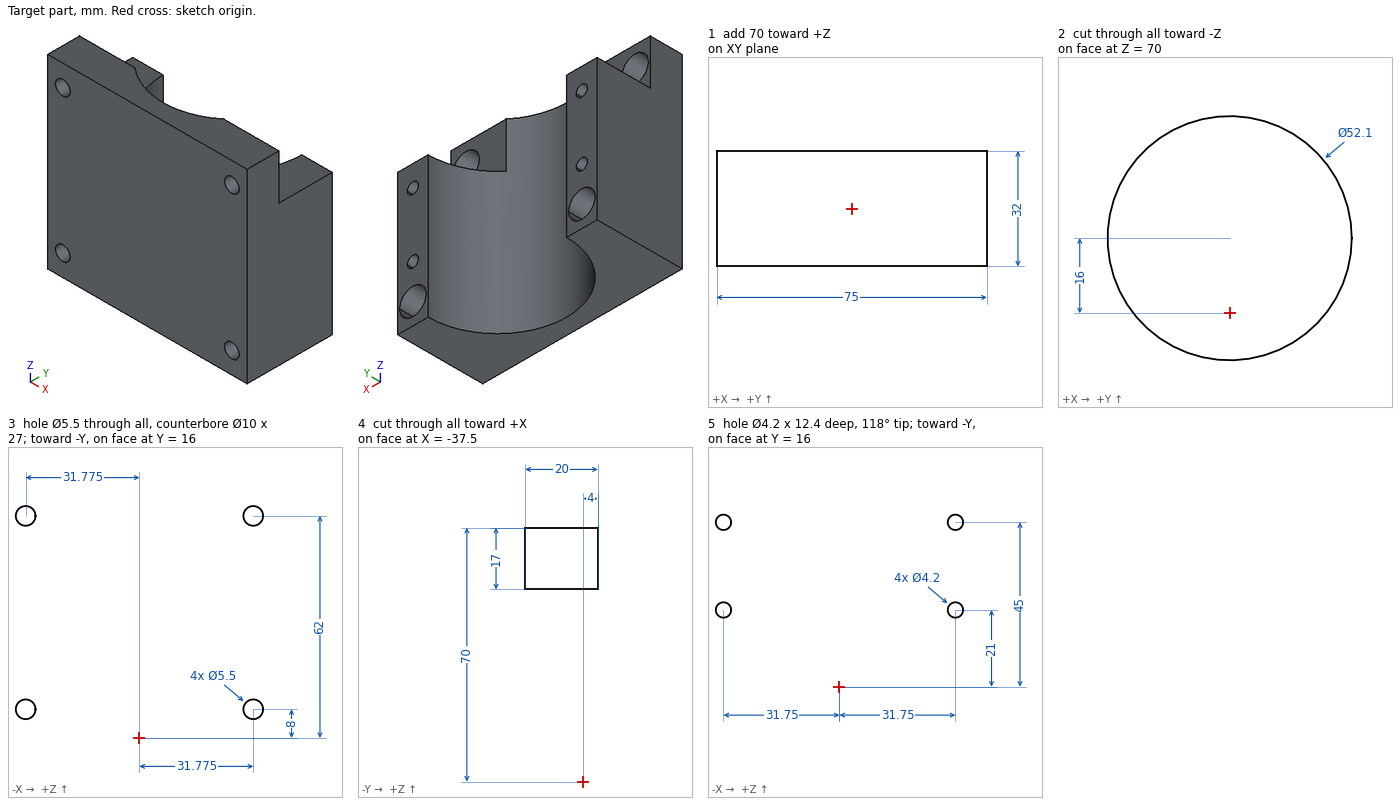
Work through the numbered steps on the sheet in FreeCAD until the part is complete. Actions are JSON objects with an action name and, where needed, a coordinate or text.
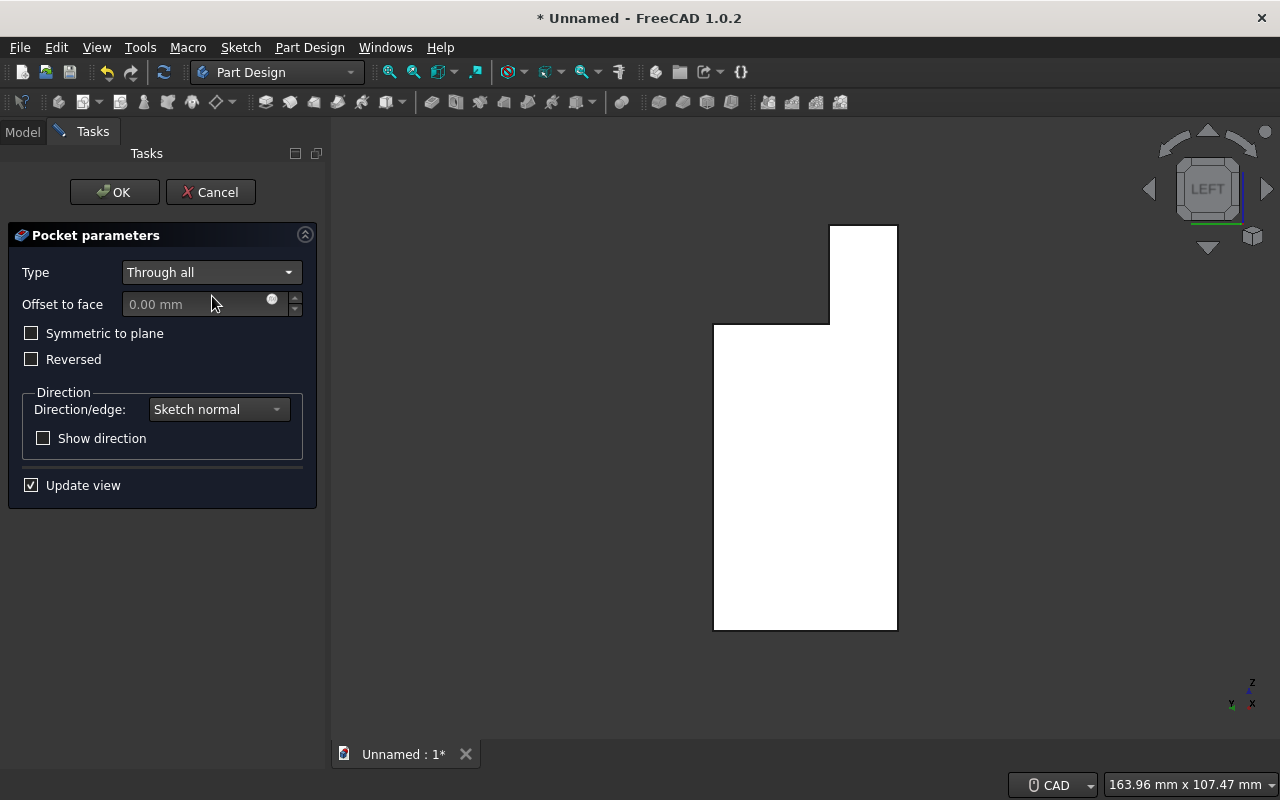
{"action": "left_click", "coordinate": [115, 192]}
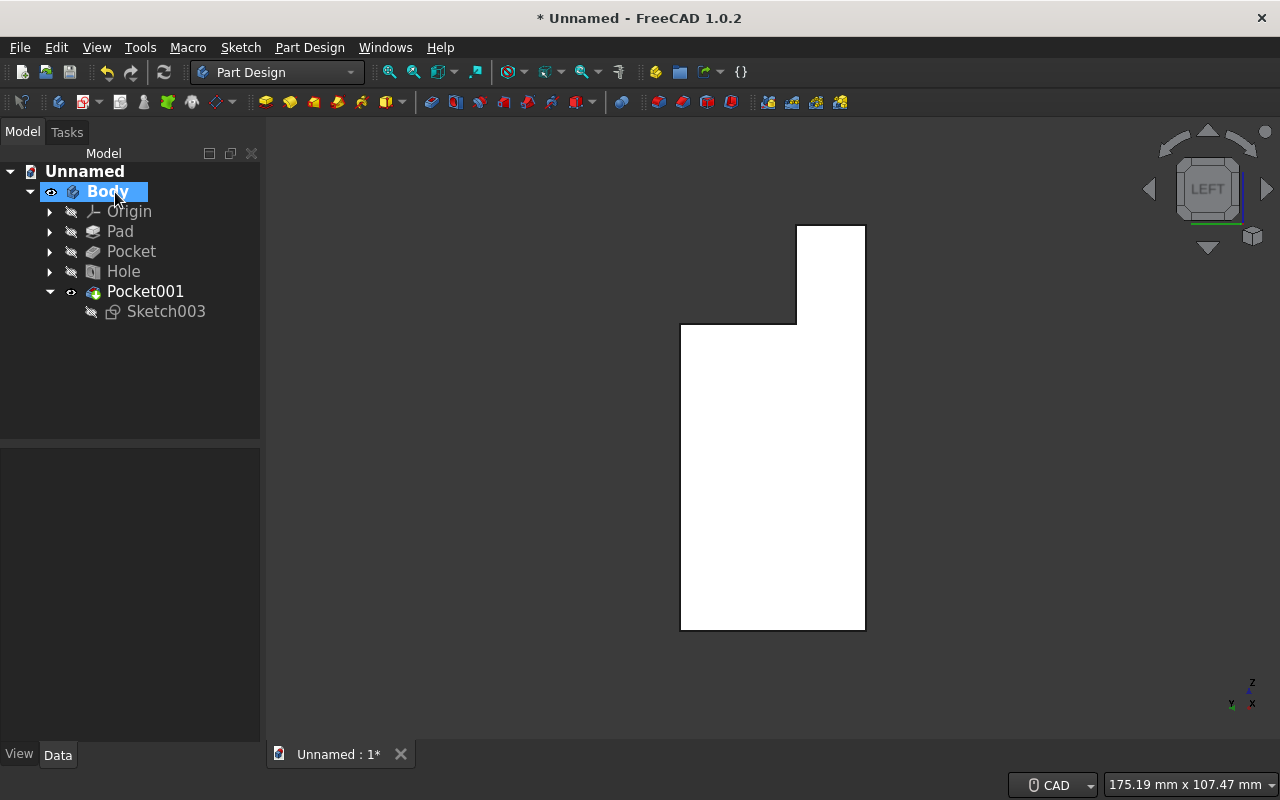
{"action": "key", "text": "4"}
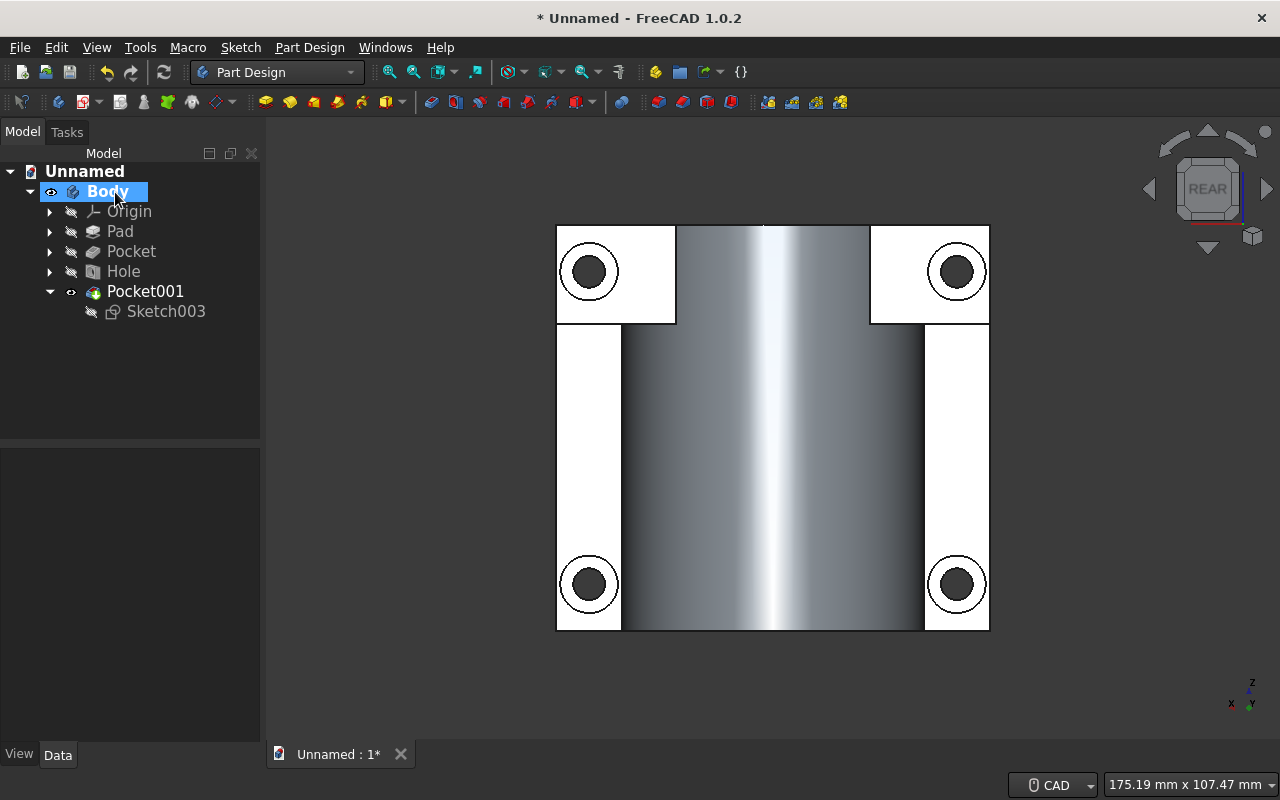
{"action": "left_click", "coordinate": [957, 389]}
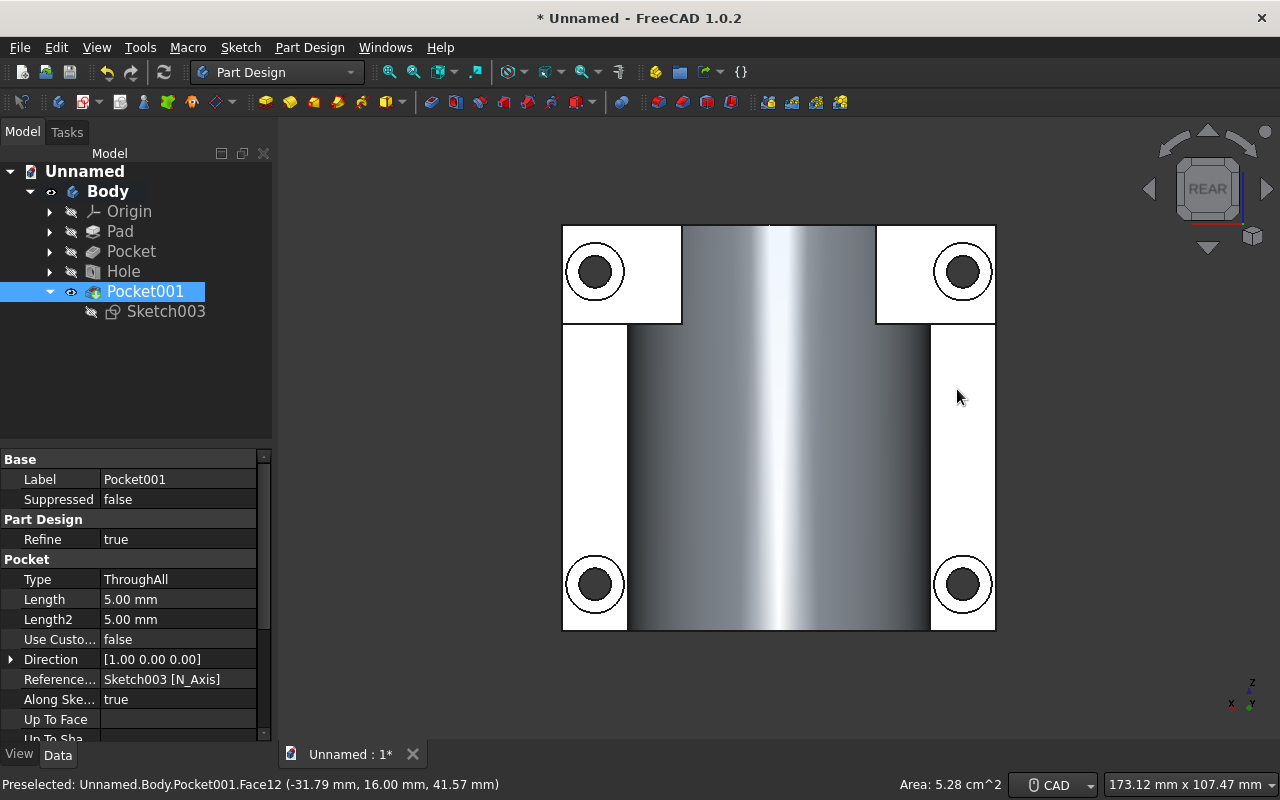
{"action": "left_click", "coordinate": [84, 102]}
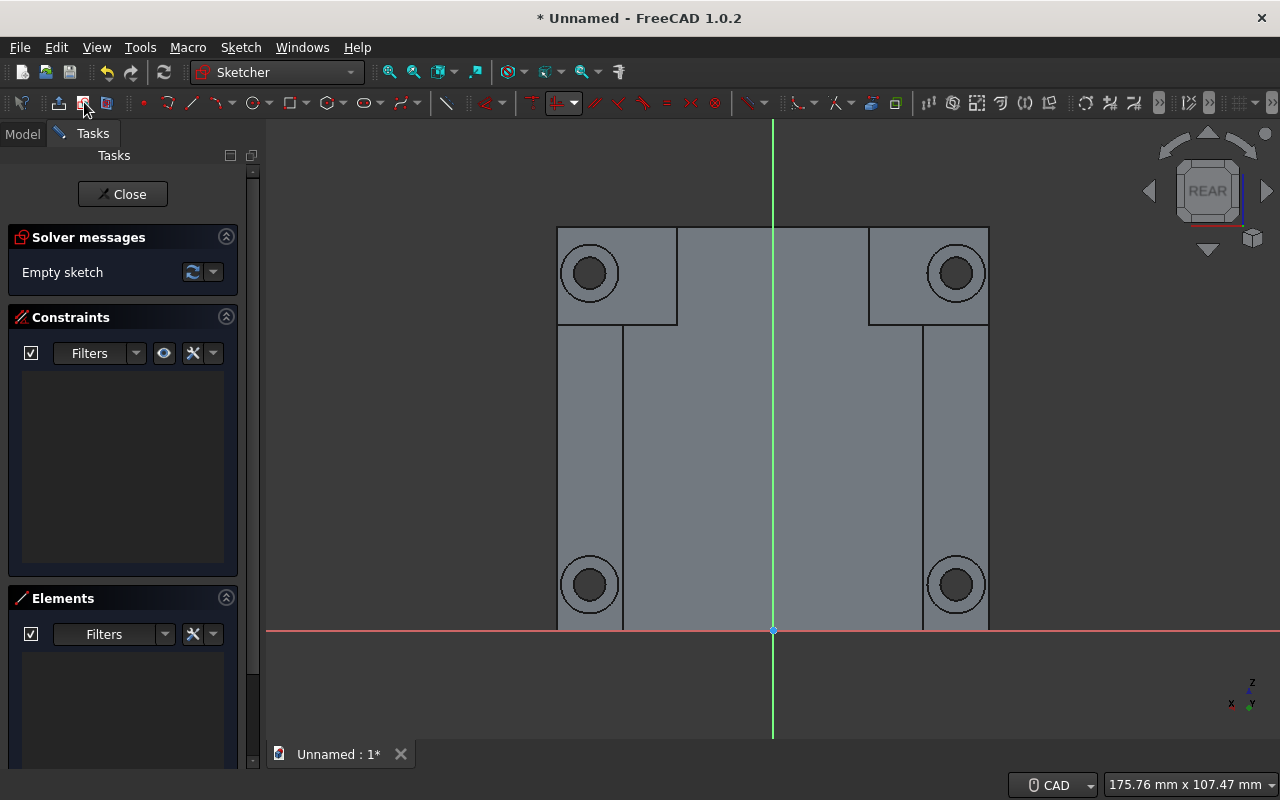
{"action": "scroll", "coordinate": [912, 629], "scroll_direction": "up", "scroll_amount": 2}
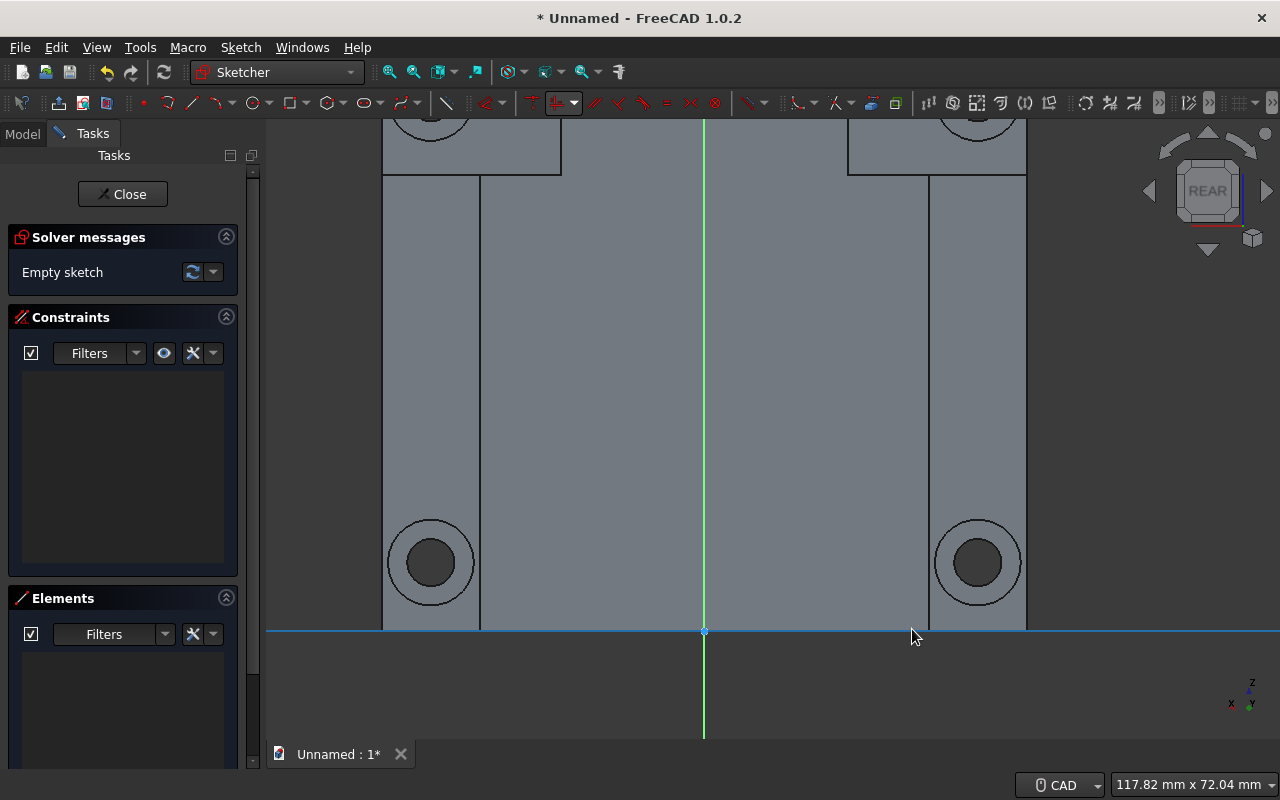
{"action": "left_click", "coordinate": [254, 104]}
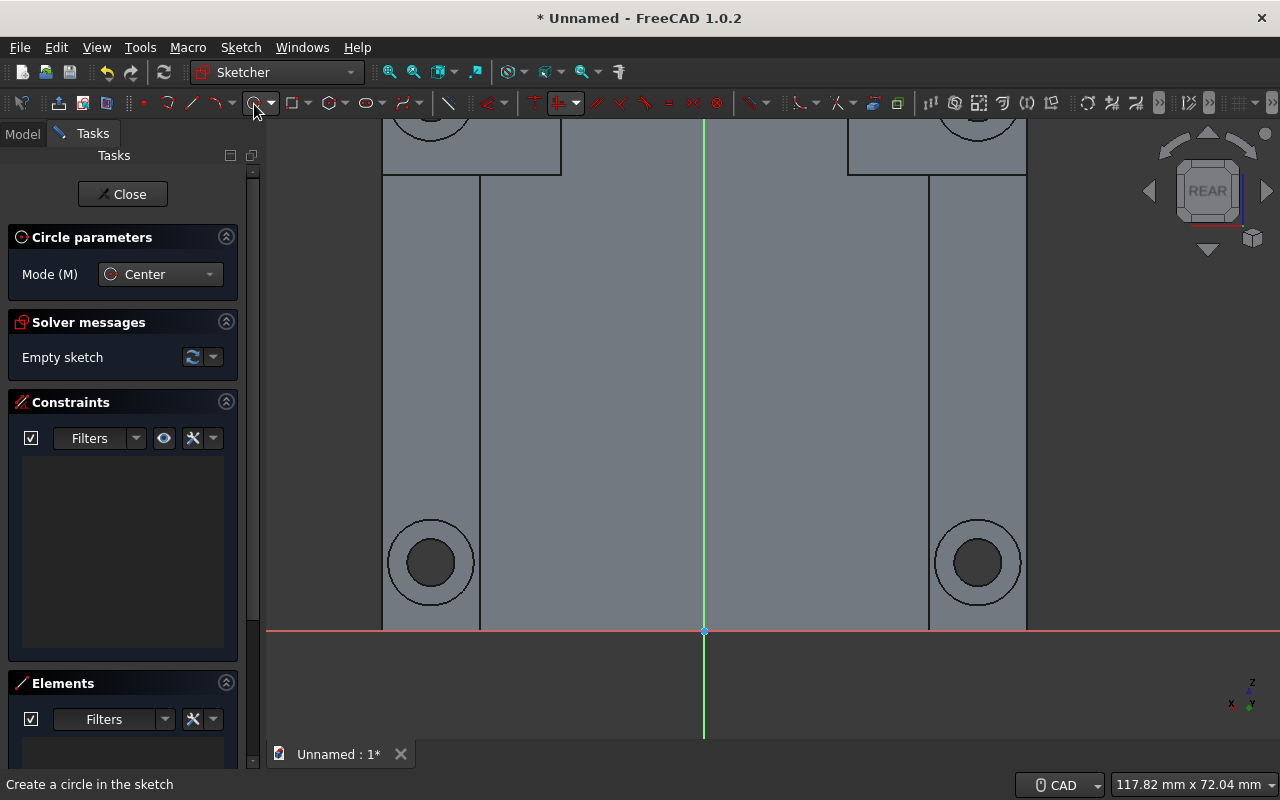
{"action": "scroll", "coordinate": [978, 451], "scroll_direction": "up", "scroll_amount": 2}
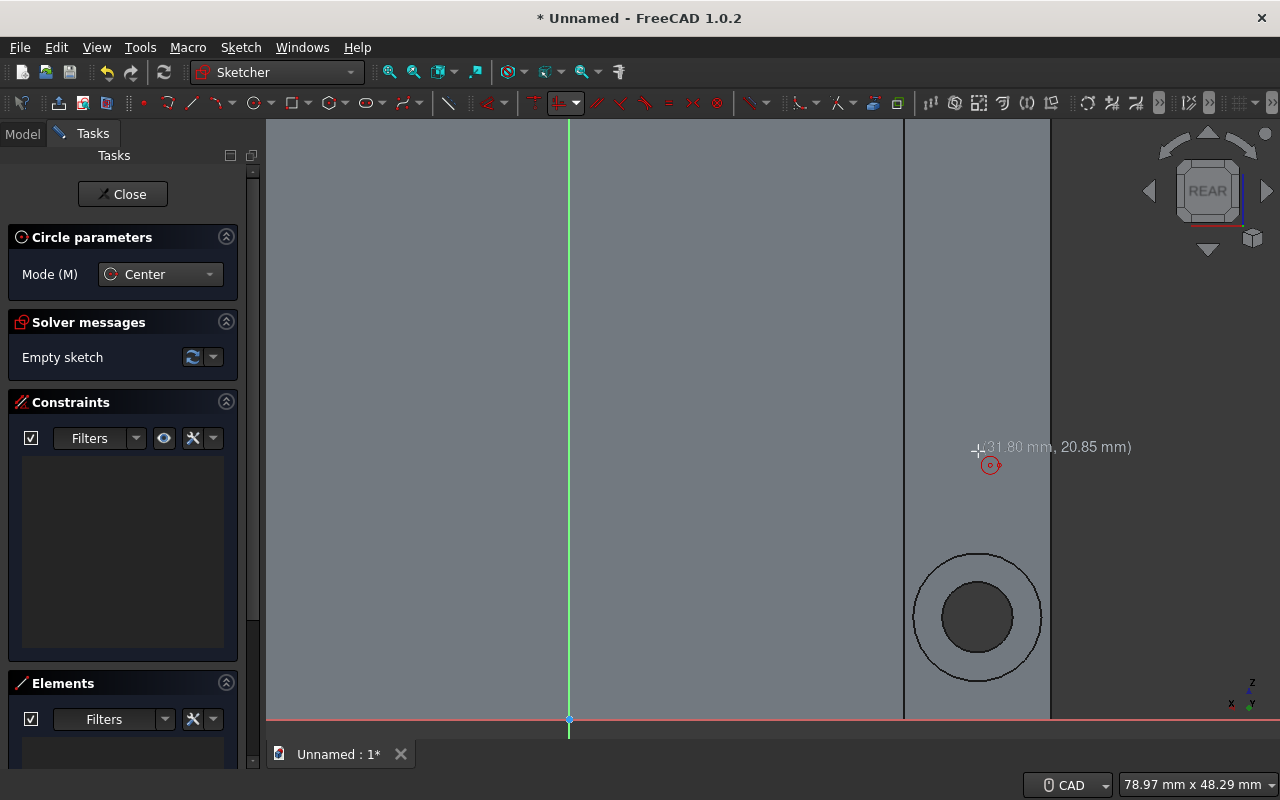
{"action": "left_click", "coordinate": [977, 450]}
{"action": "left_click", "coordinate": [996, 431]}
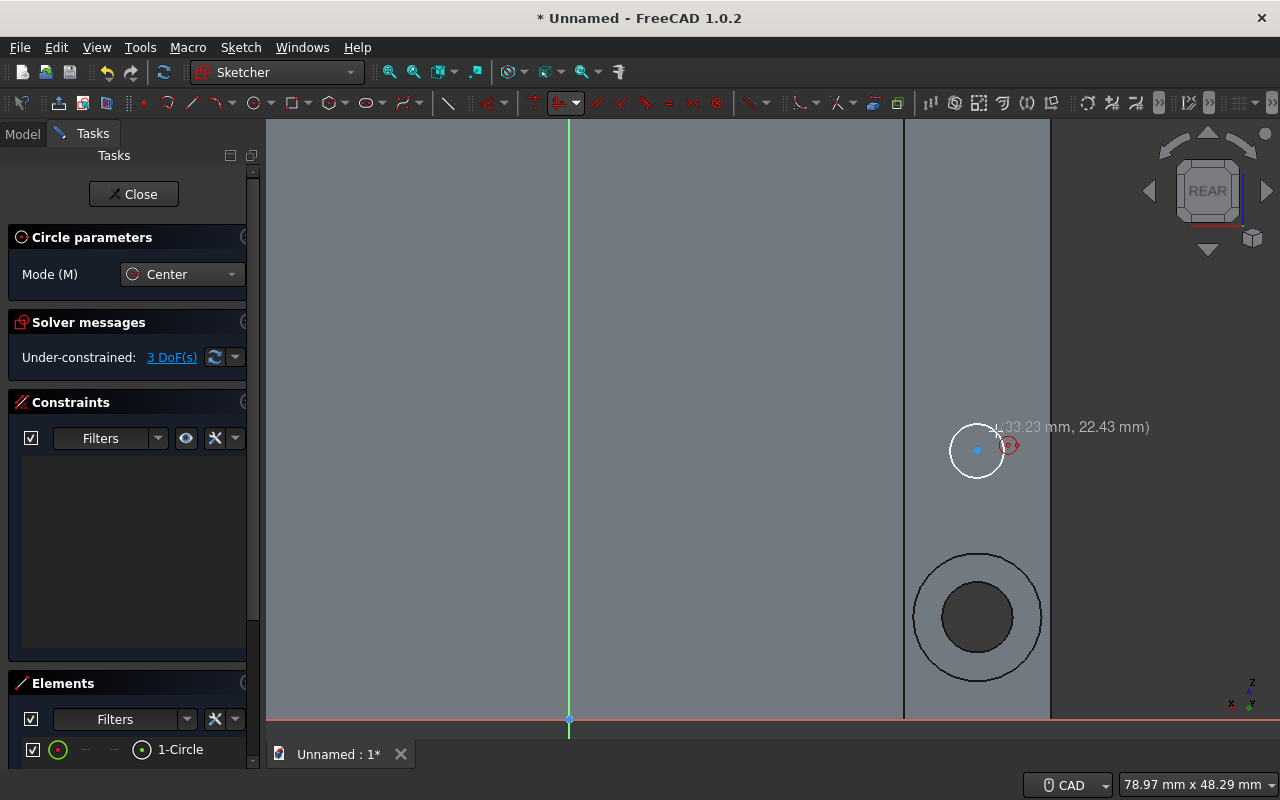
{"action": "scroll", "coordinate": [979, 452], "scroll_direction": "down", "scroll_amount": 2}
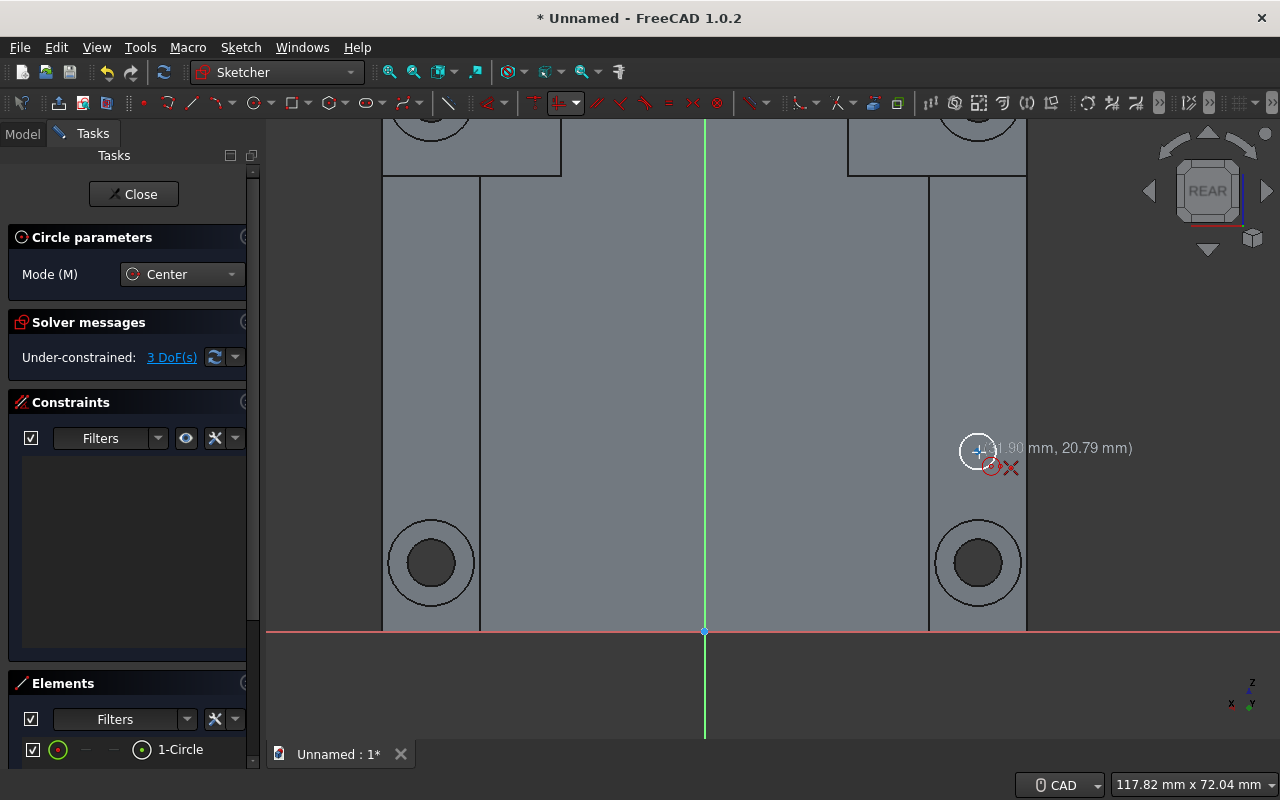
{"action": "scroll", "coordinate": [978, 244], "scroll_direction": "up", "scroll_amount": 2}